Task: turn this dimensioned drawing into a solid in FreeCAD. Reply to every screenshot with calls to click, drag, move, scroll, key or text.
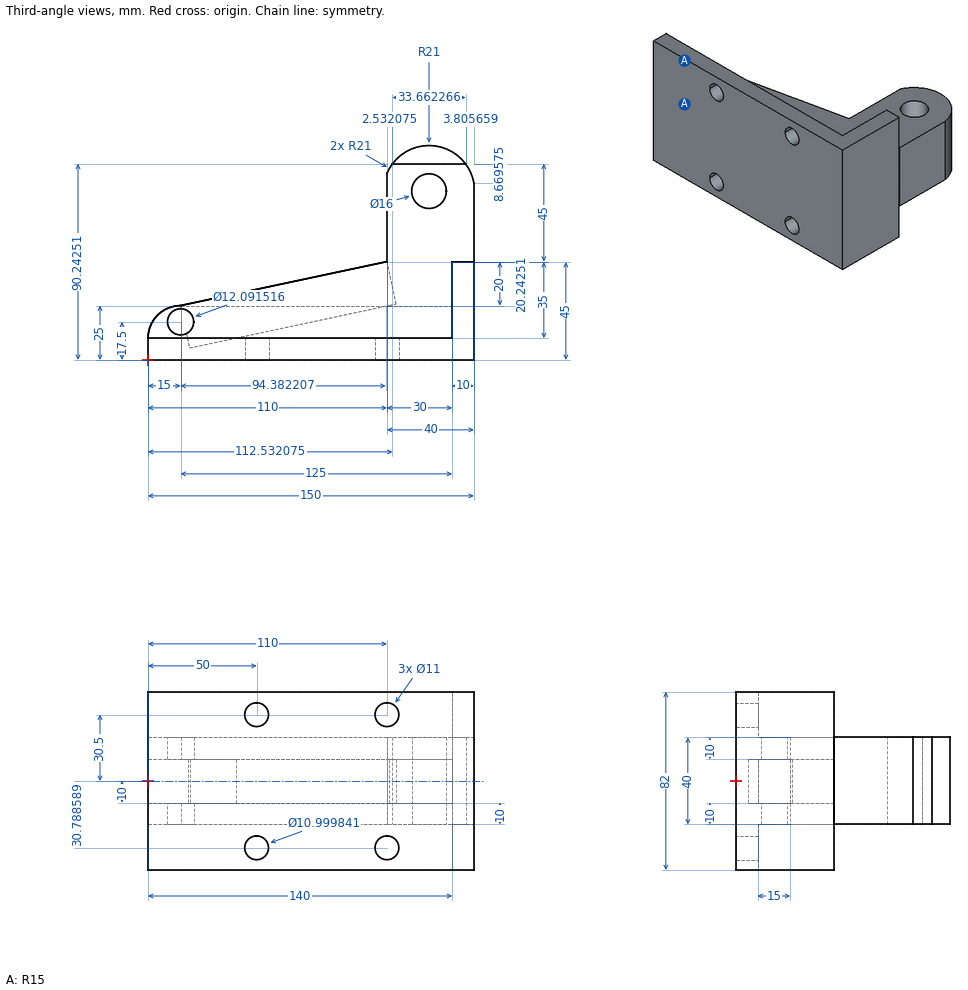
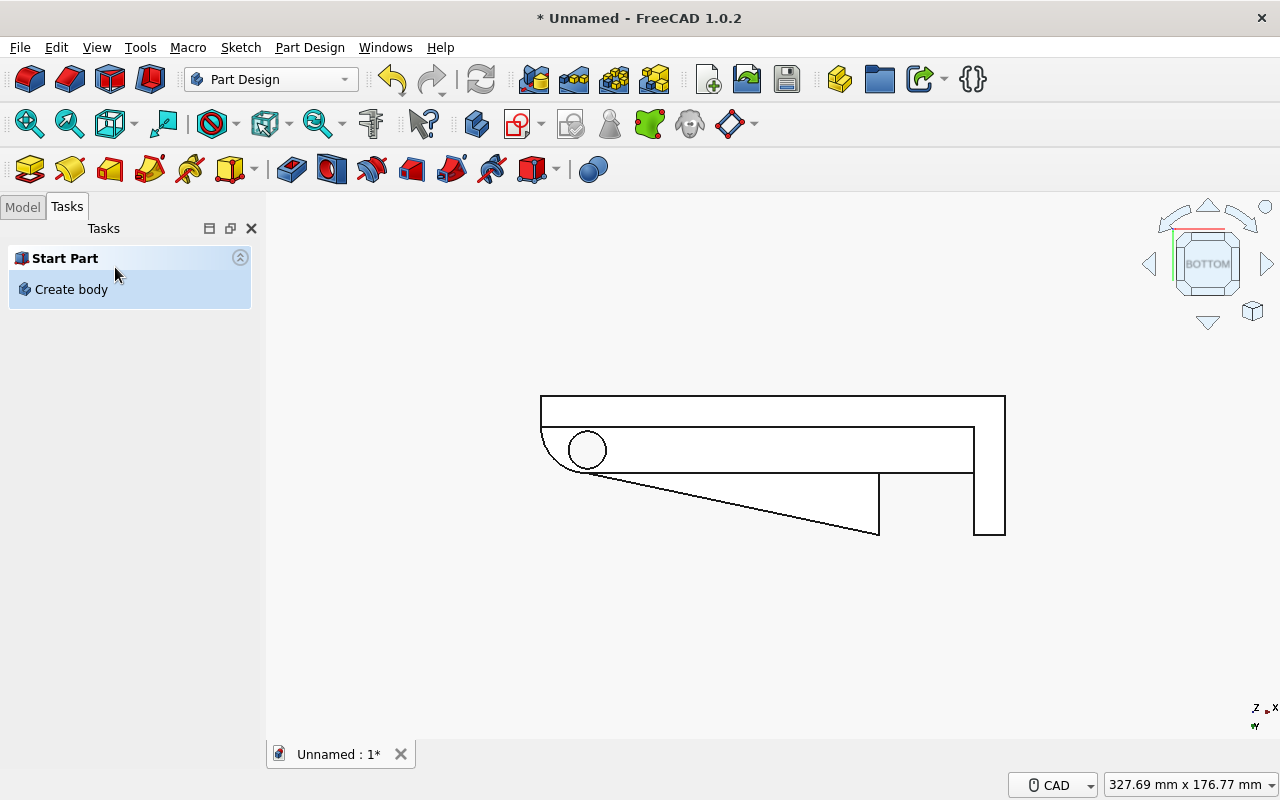
click(943, 449)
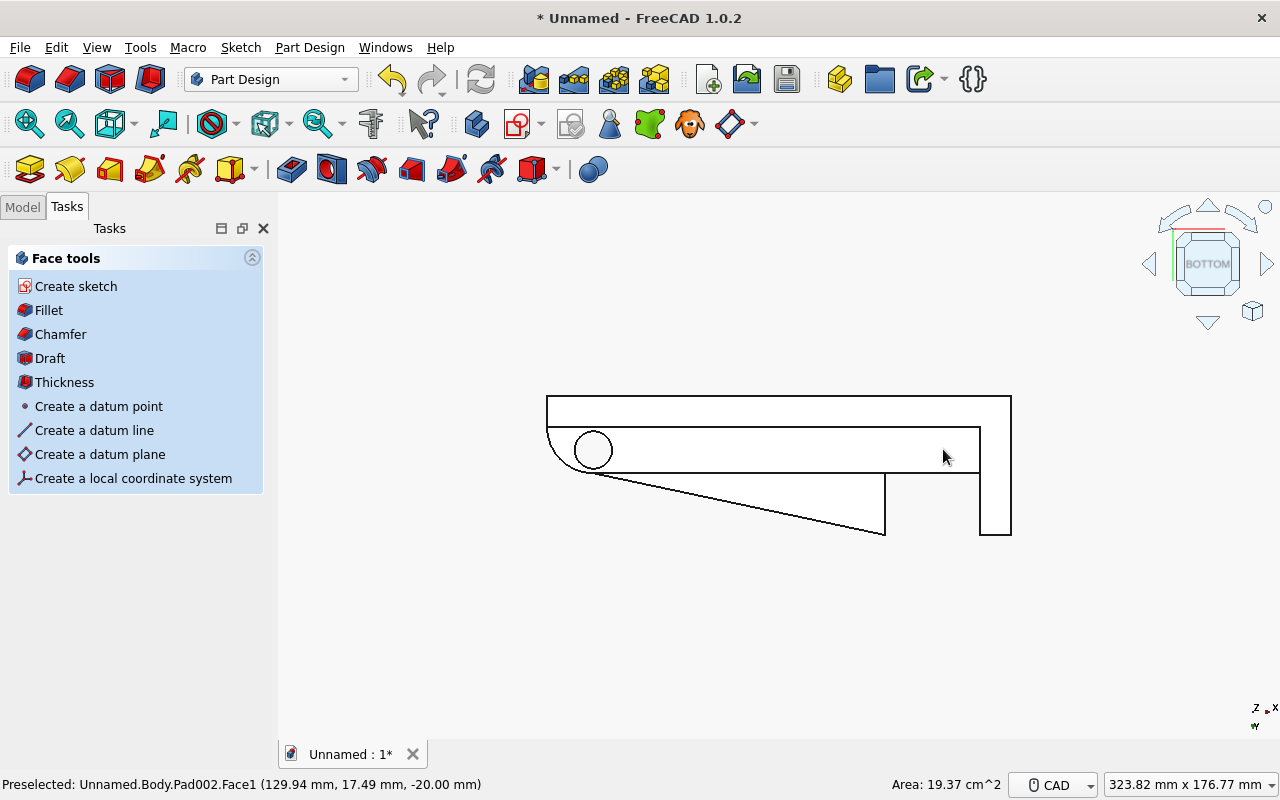
click(518, 124)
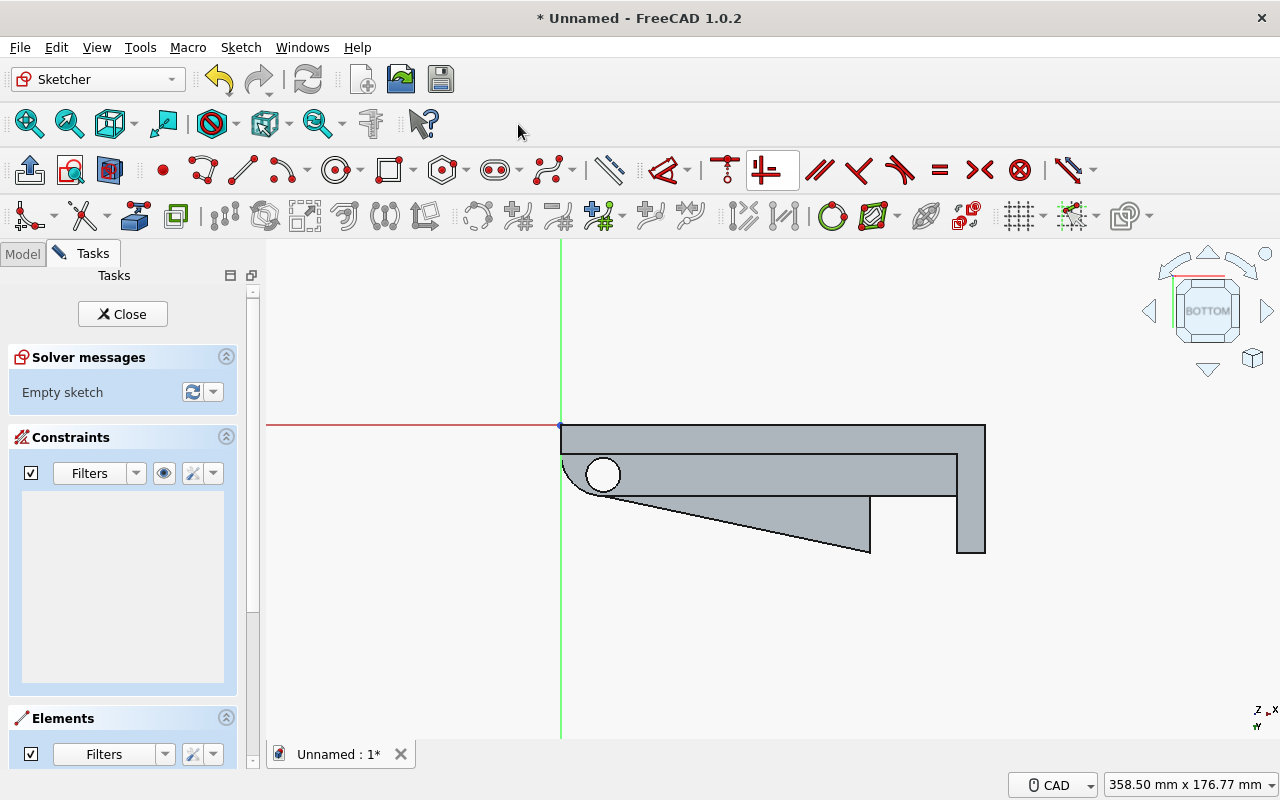
key(q)
key(s)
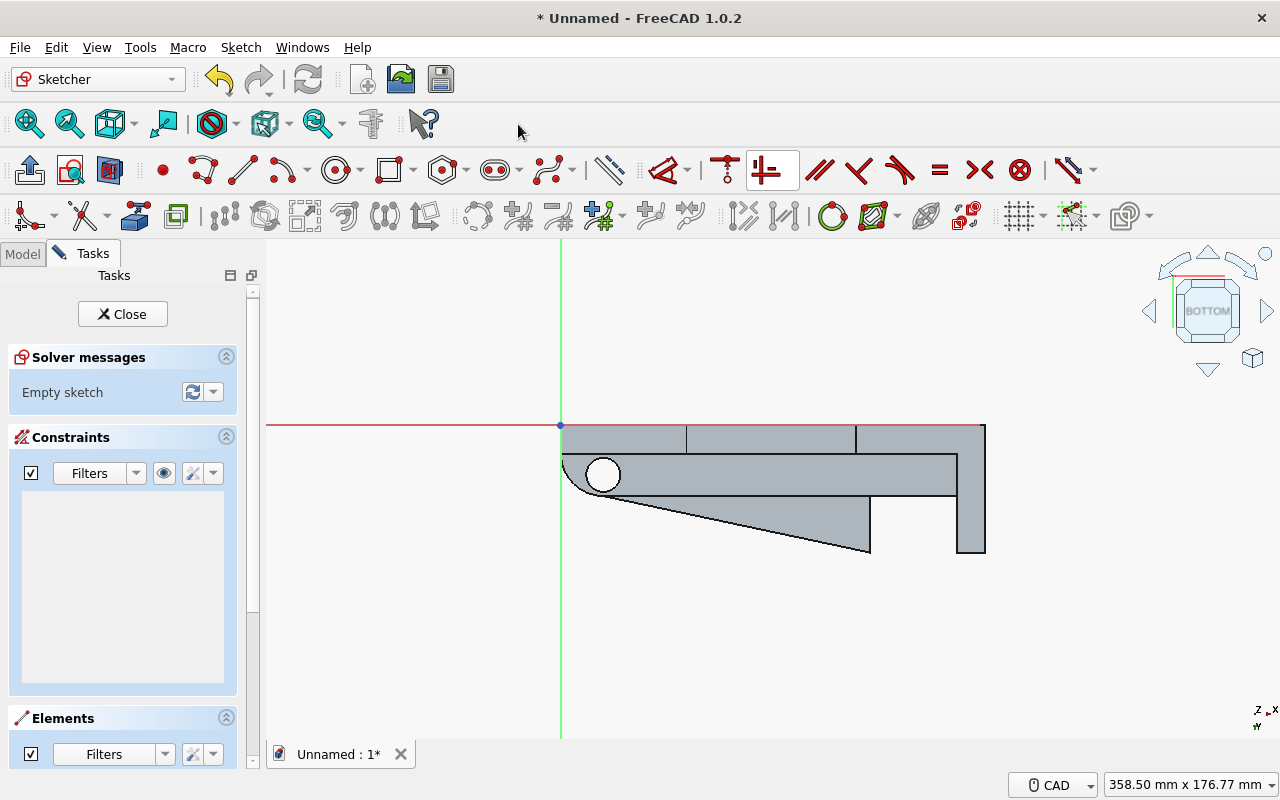
scroll(869, 490, up, 2)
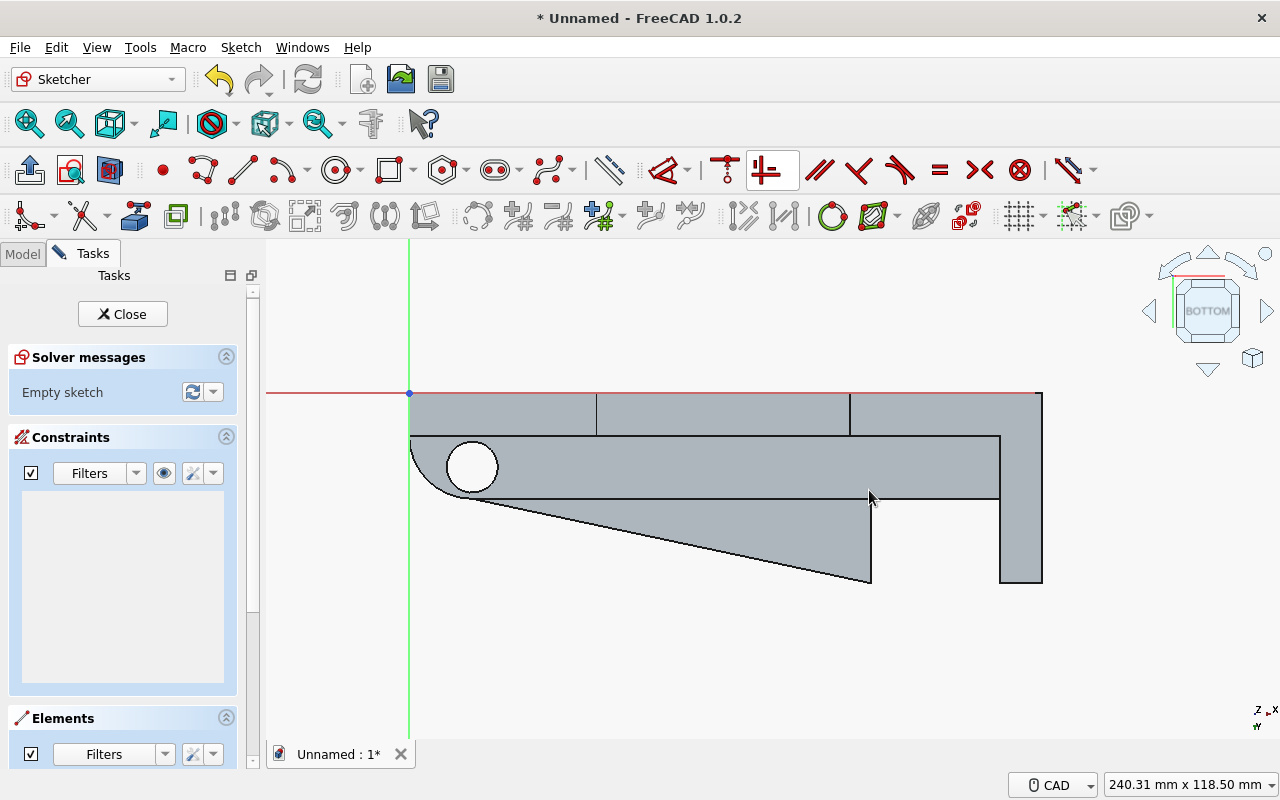
click(204, 170)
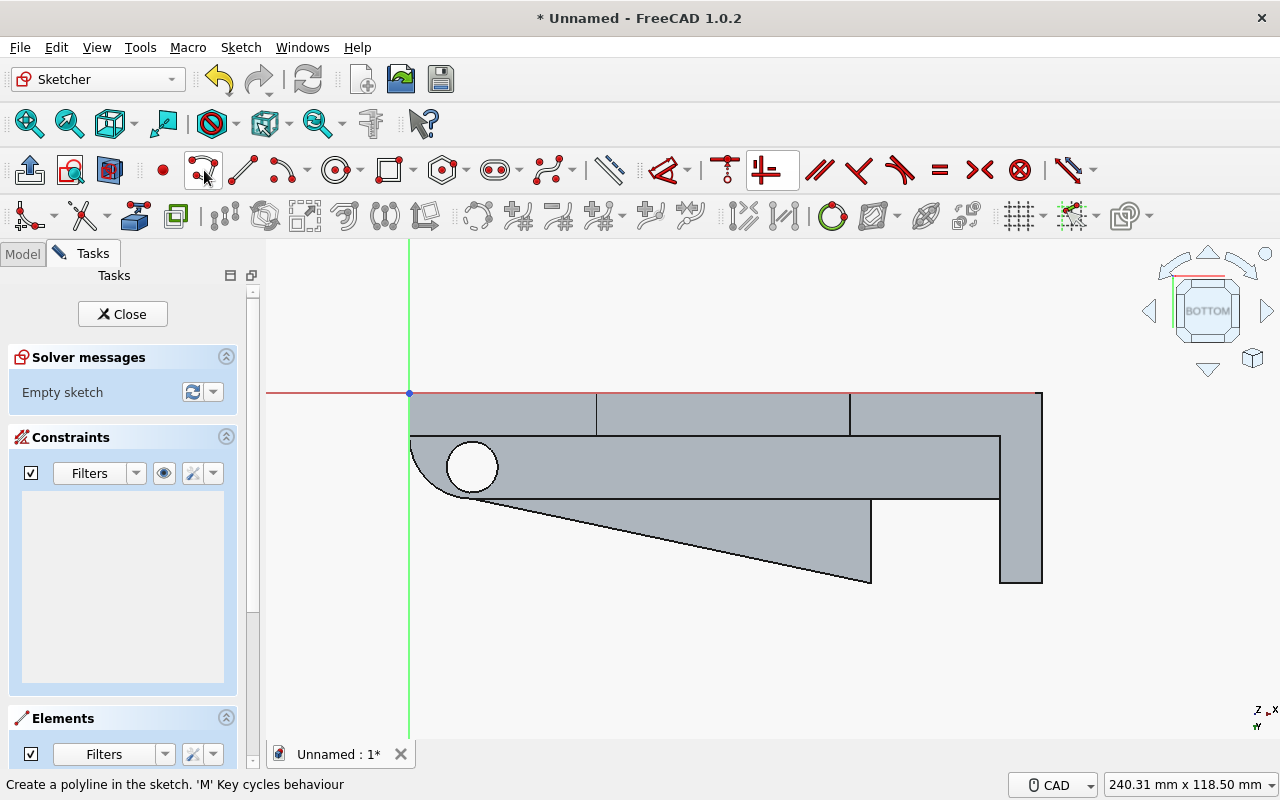
click(472, 499)
click(873, 584)
click(1000, 584)
click(1000, 499)
click(472, 500)
key(Escape)
key(Escape)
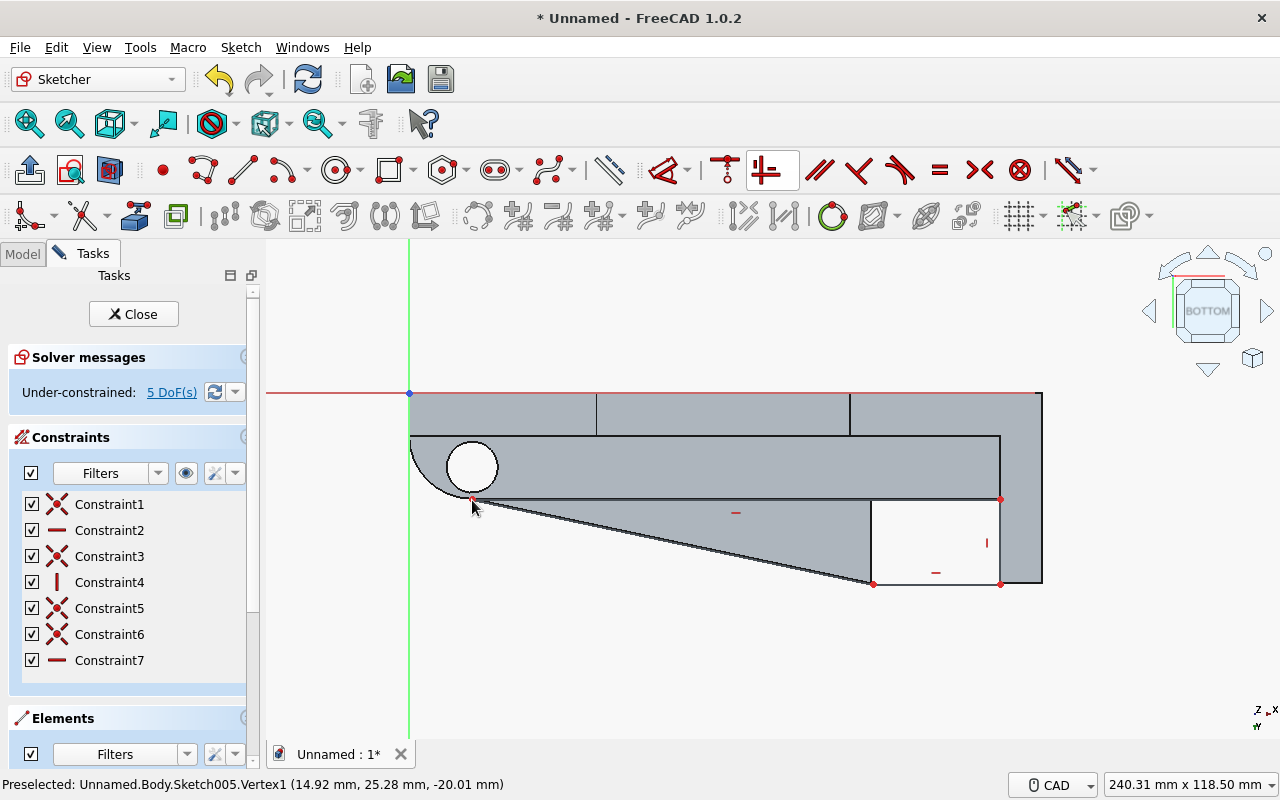
click(664, 170)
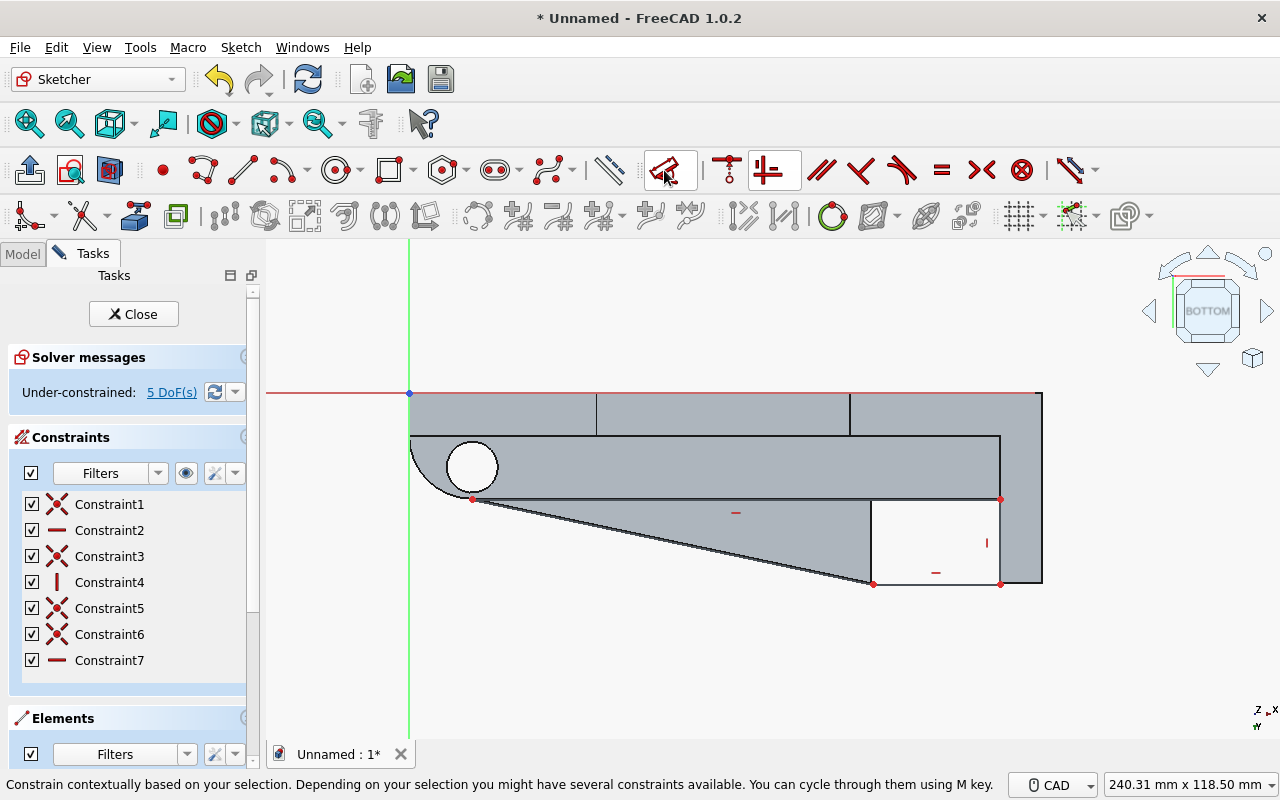
click(911, 585)
click(937, 619)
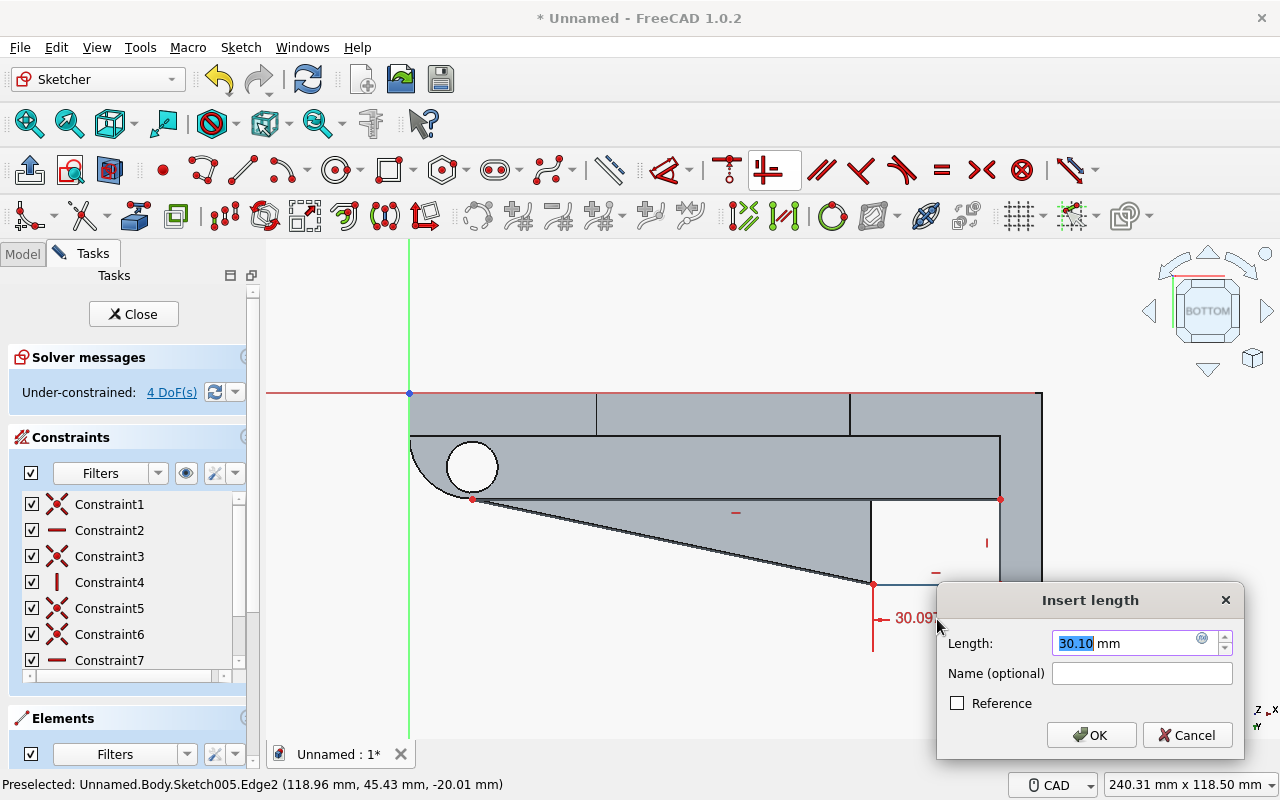
text(30)
key(Return)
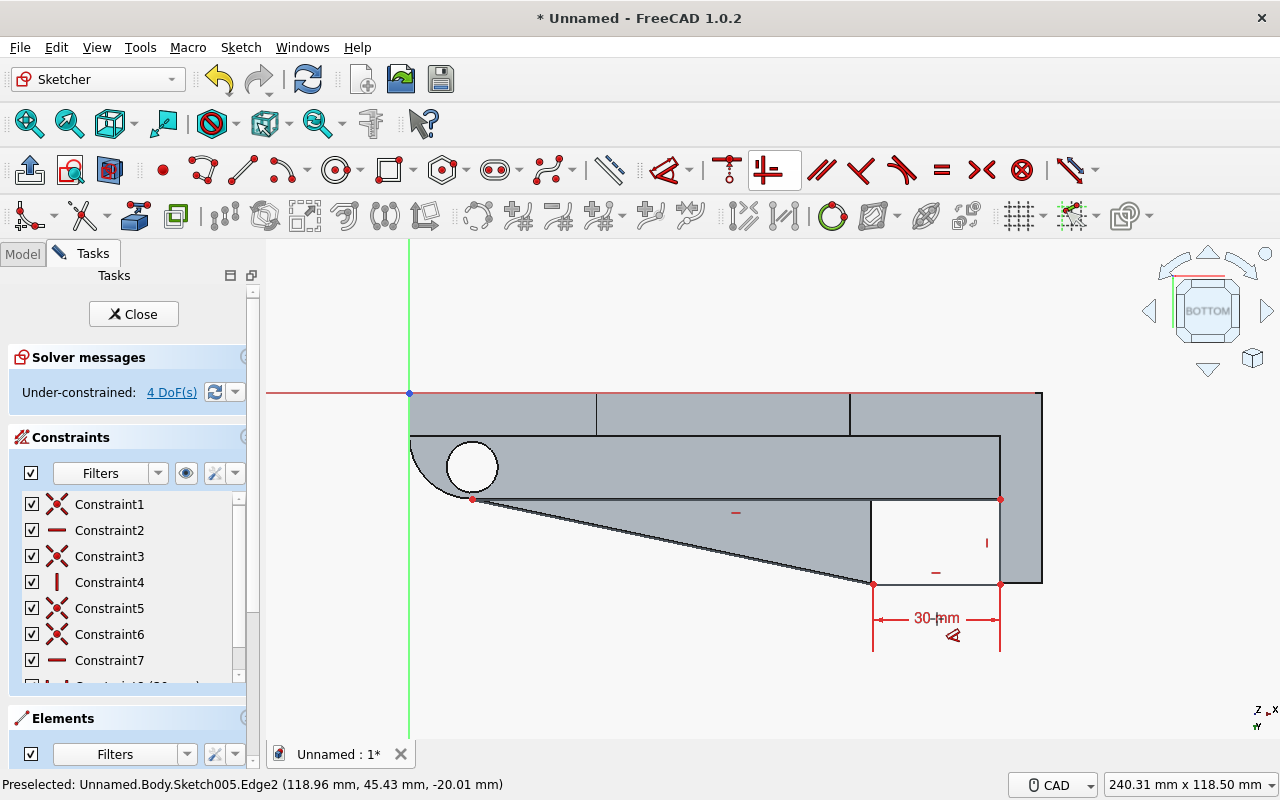
click(842, 500)
click(736, 534)